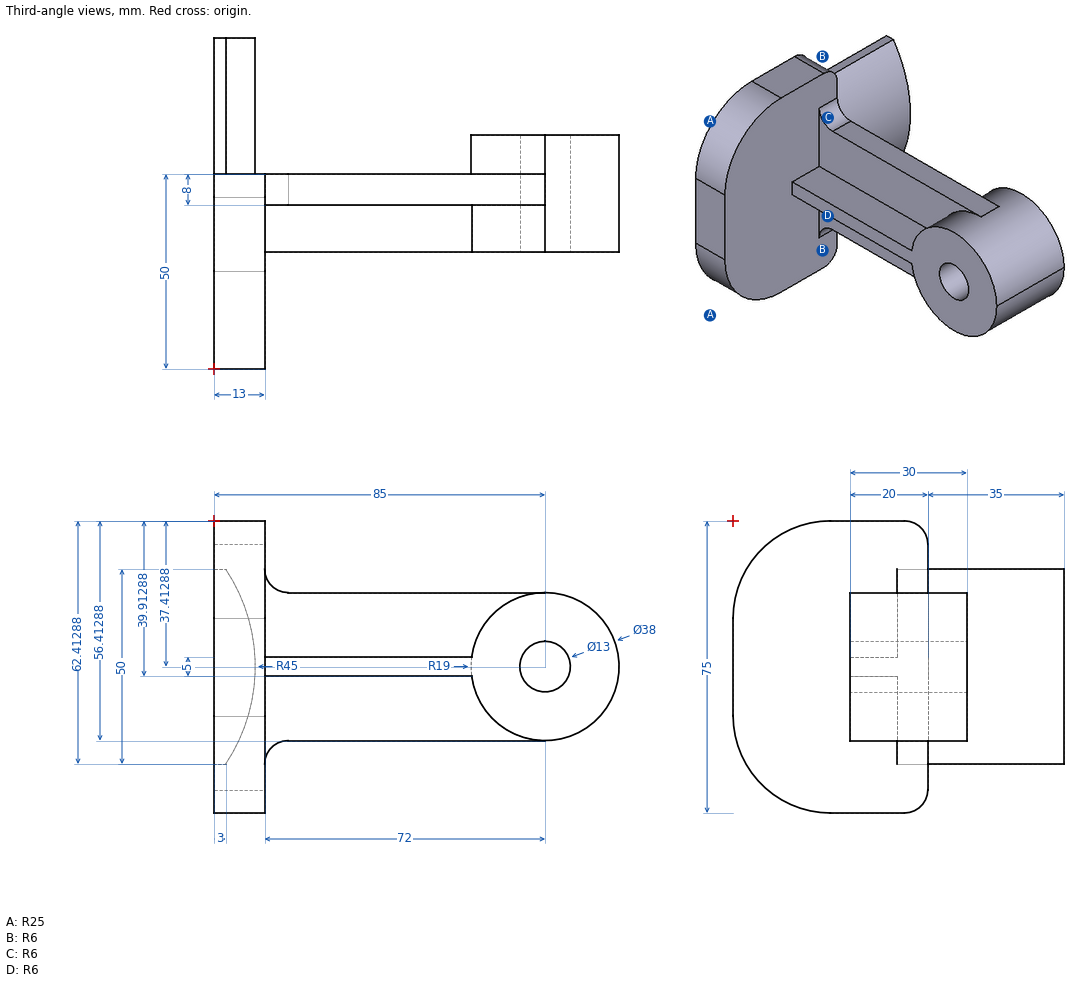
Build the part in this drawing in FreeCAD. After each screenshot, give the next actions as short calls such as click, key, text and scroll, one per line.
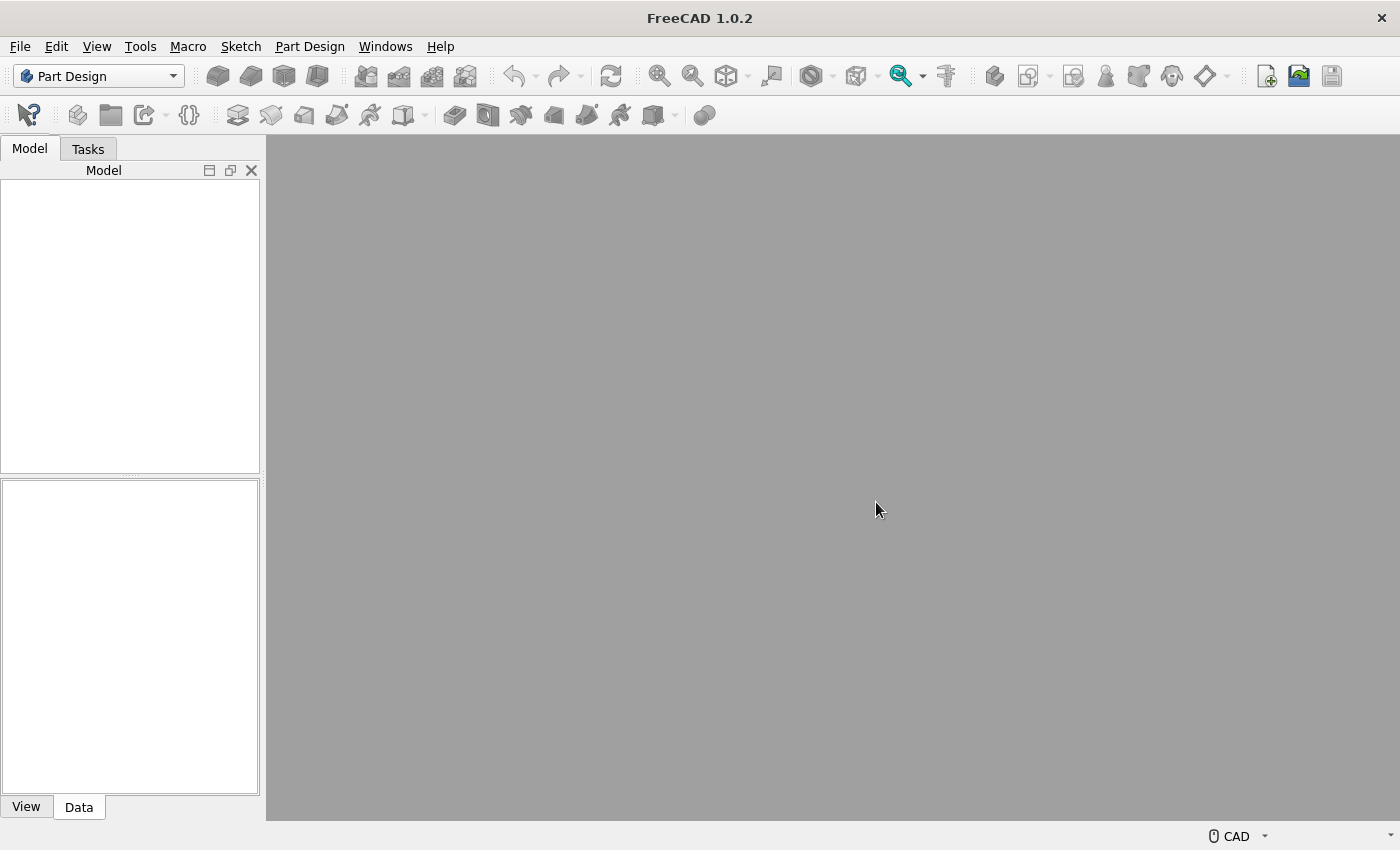
click(1266, 76)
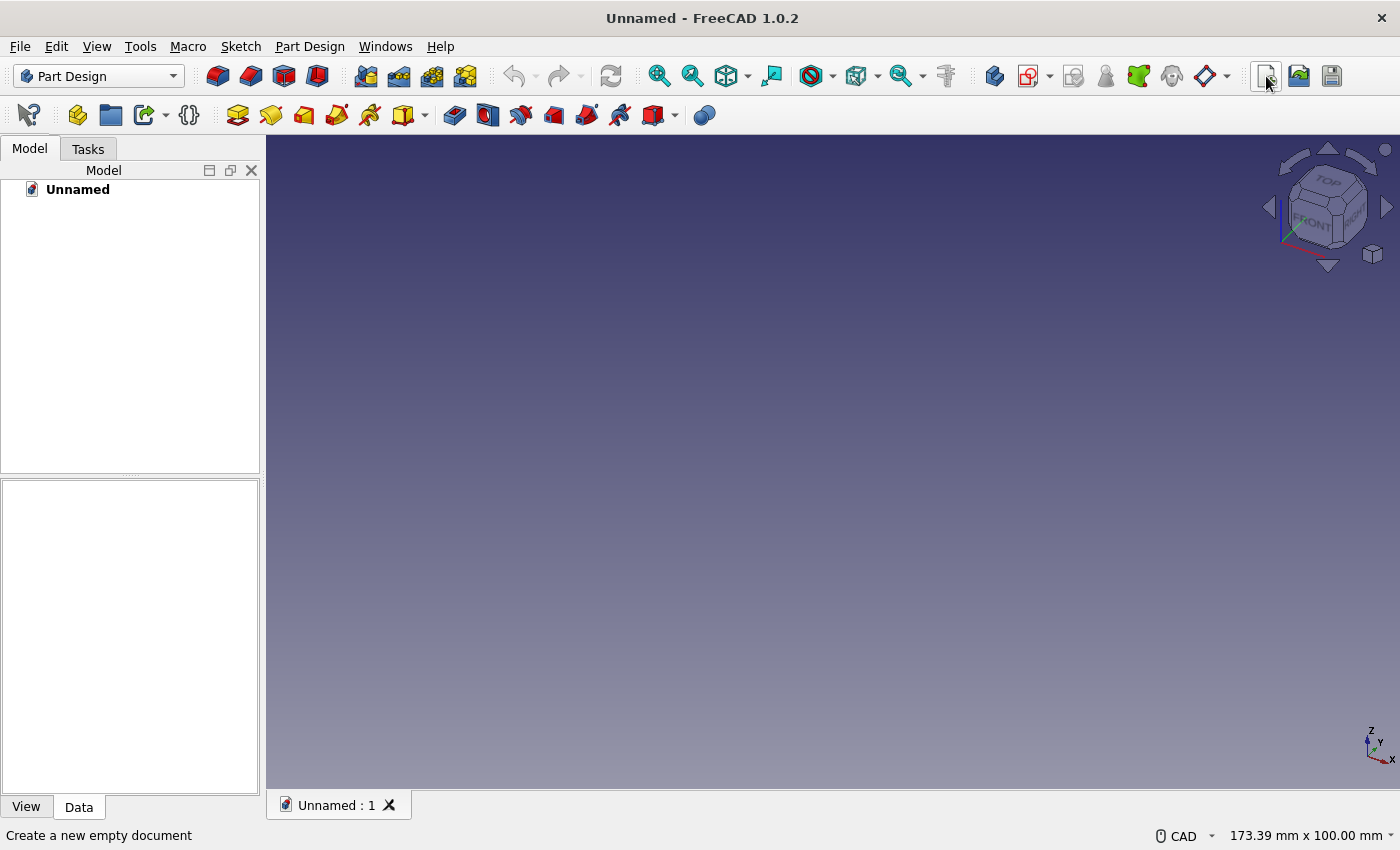
click(1028, 76)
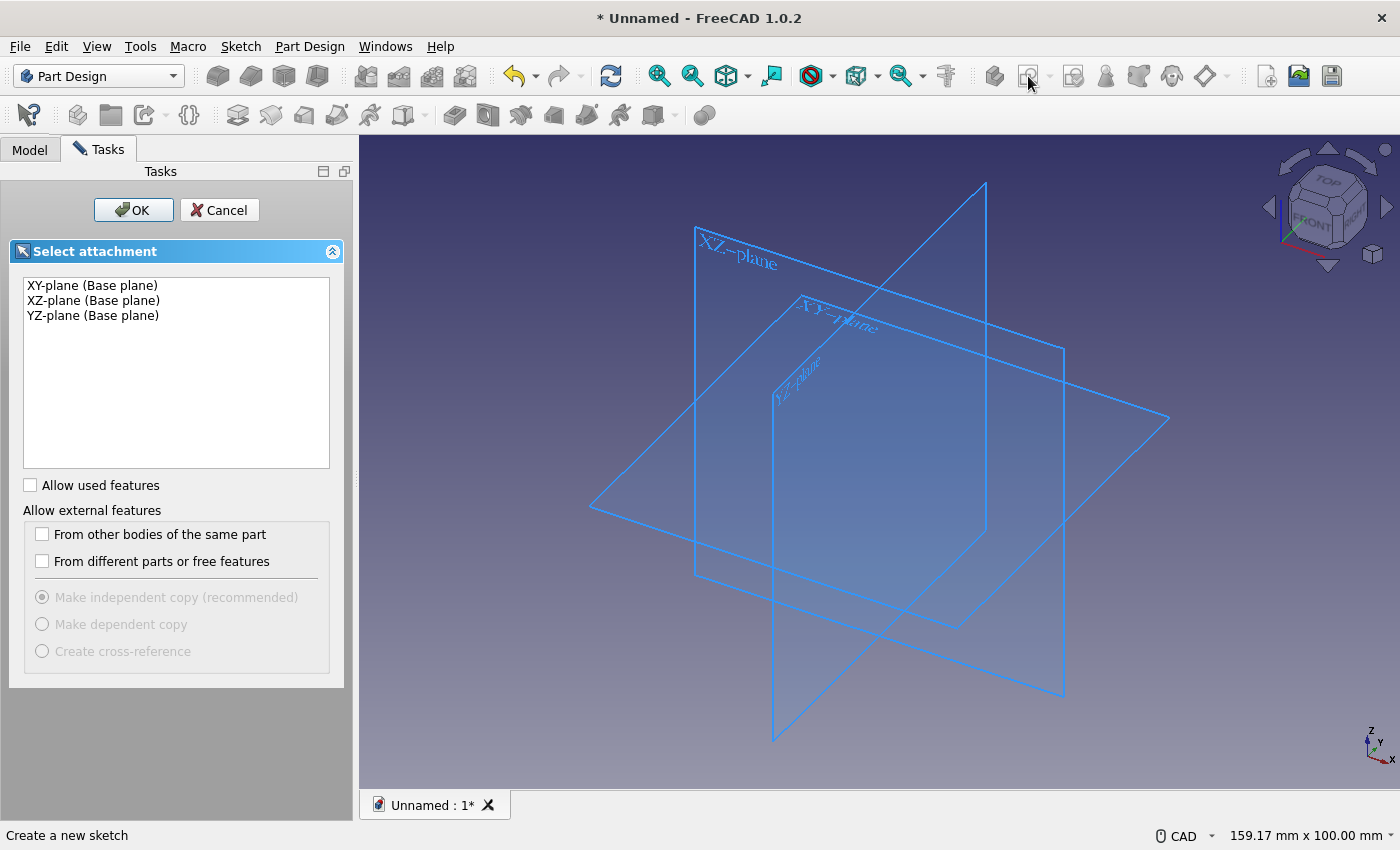
click(84, 286)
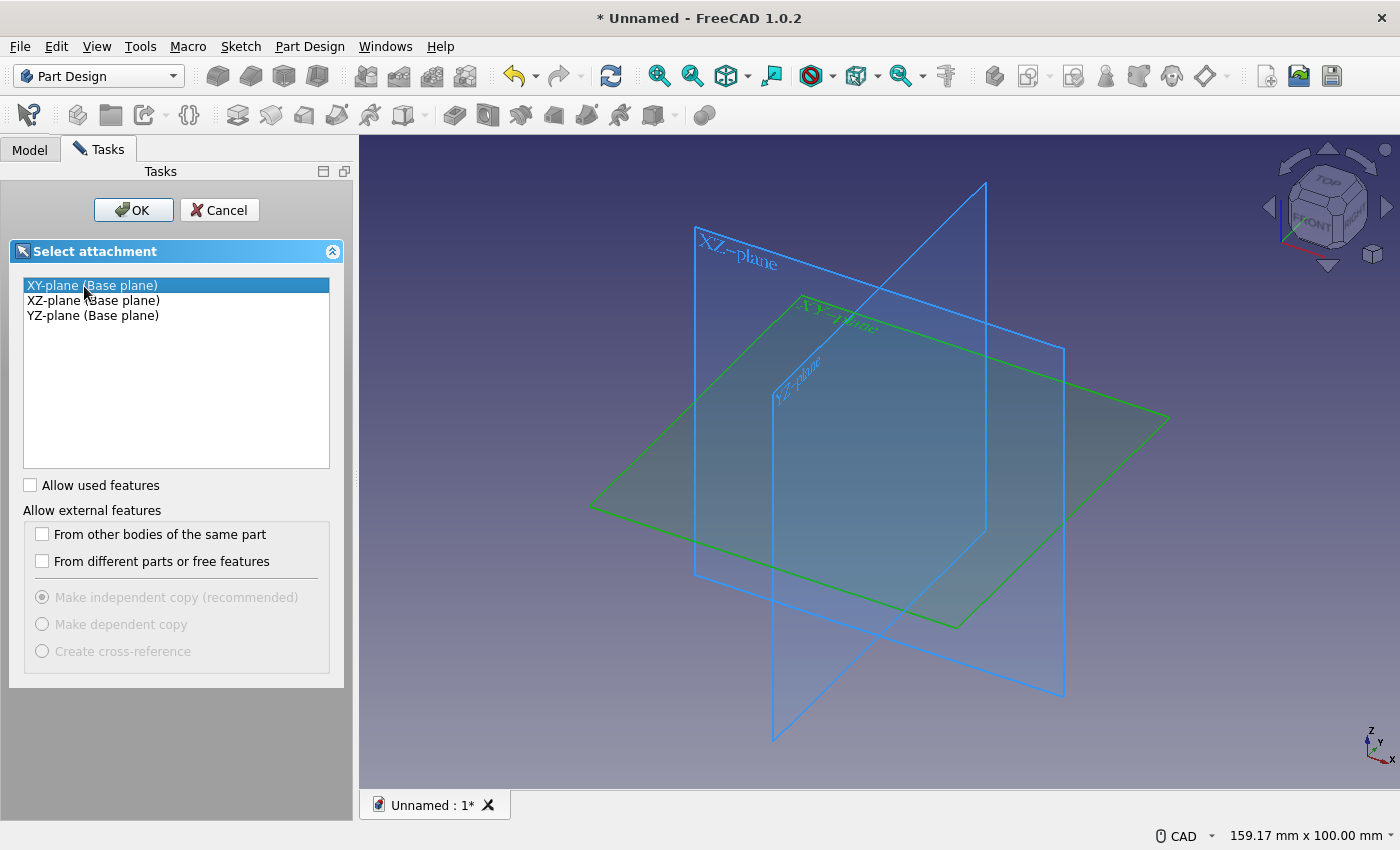
click(134, 210)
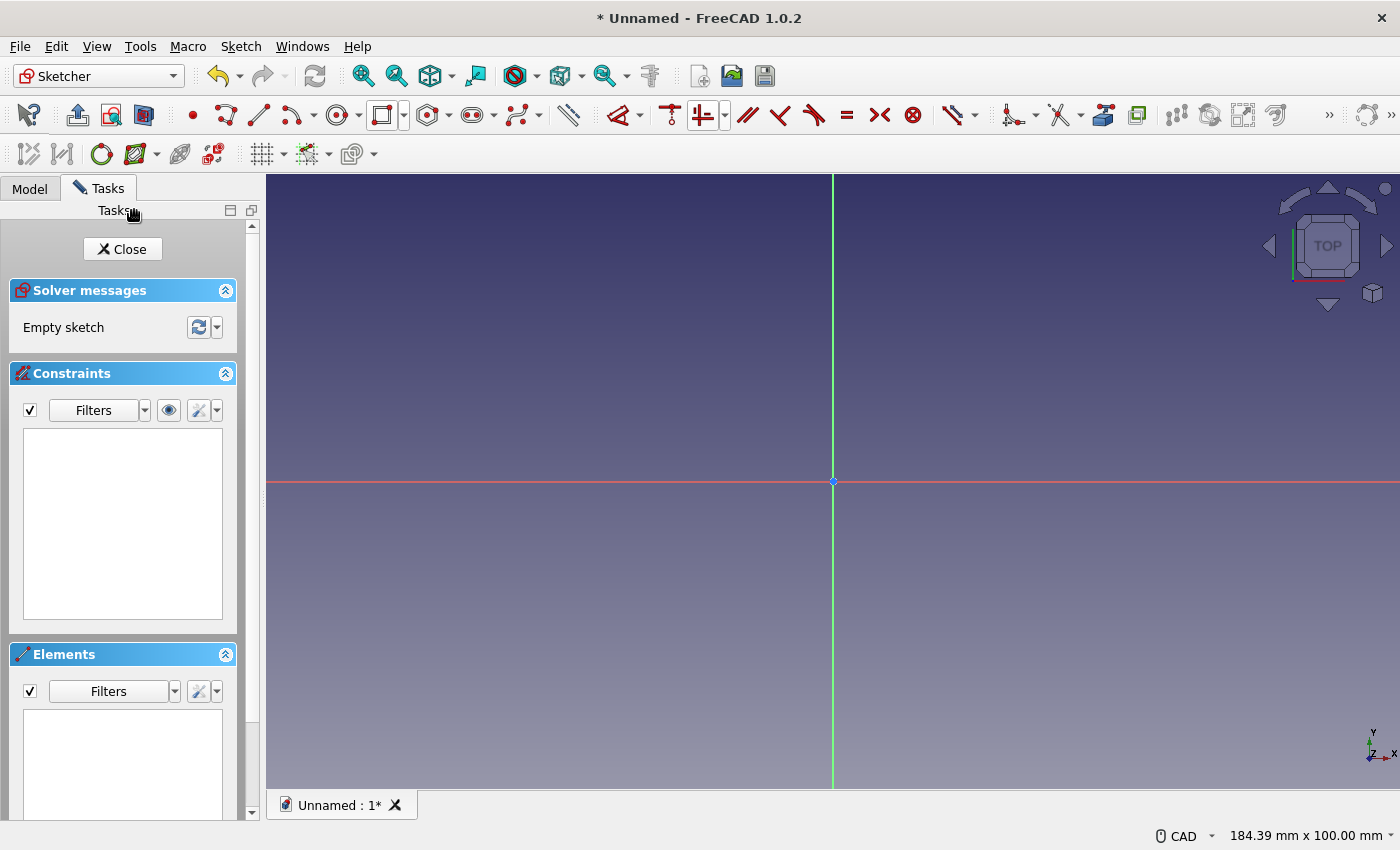
scroll(294, 761, down, 1)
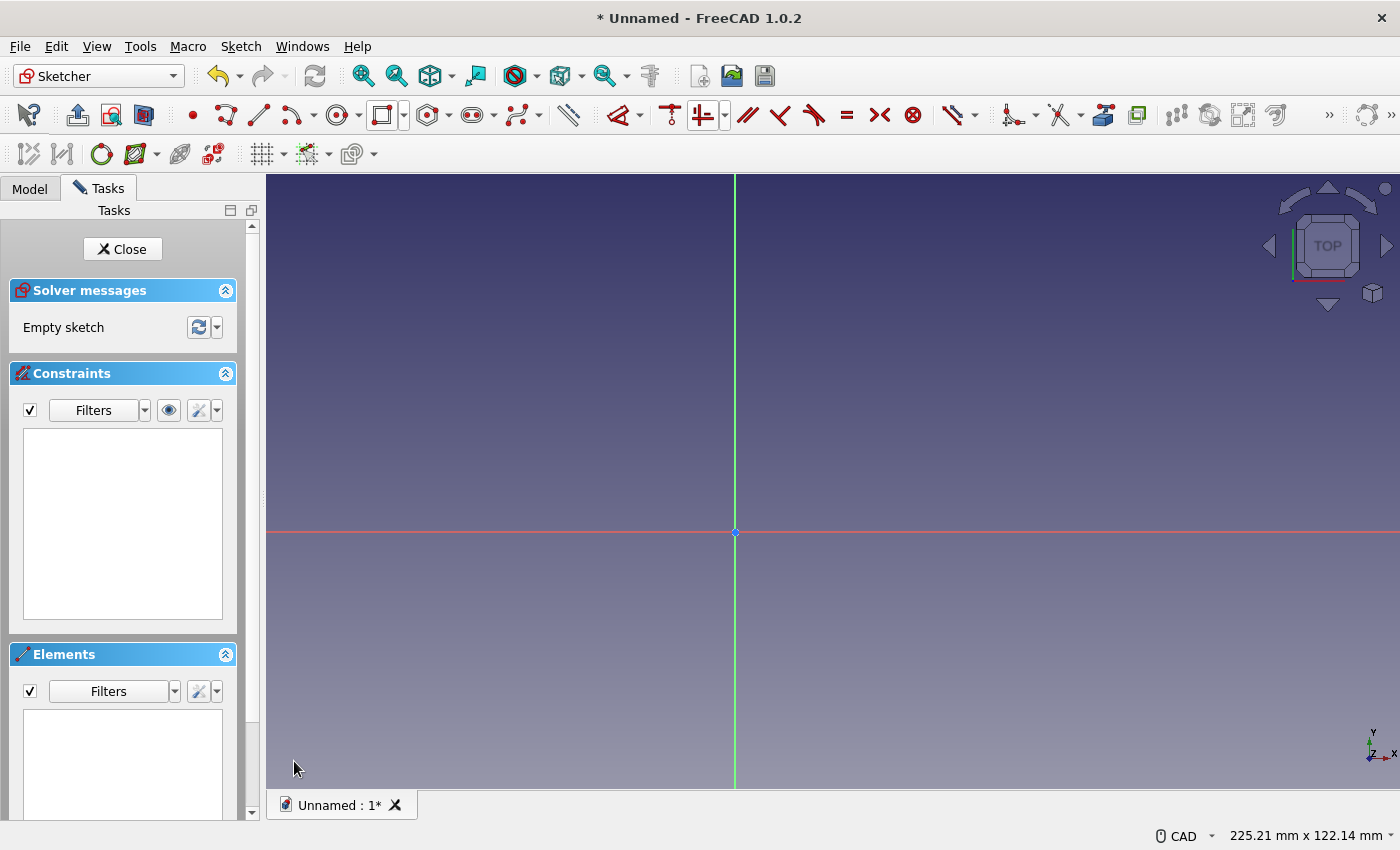
scroll(775, 254, up, 2)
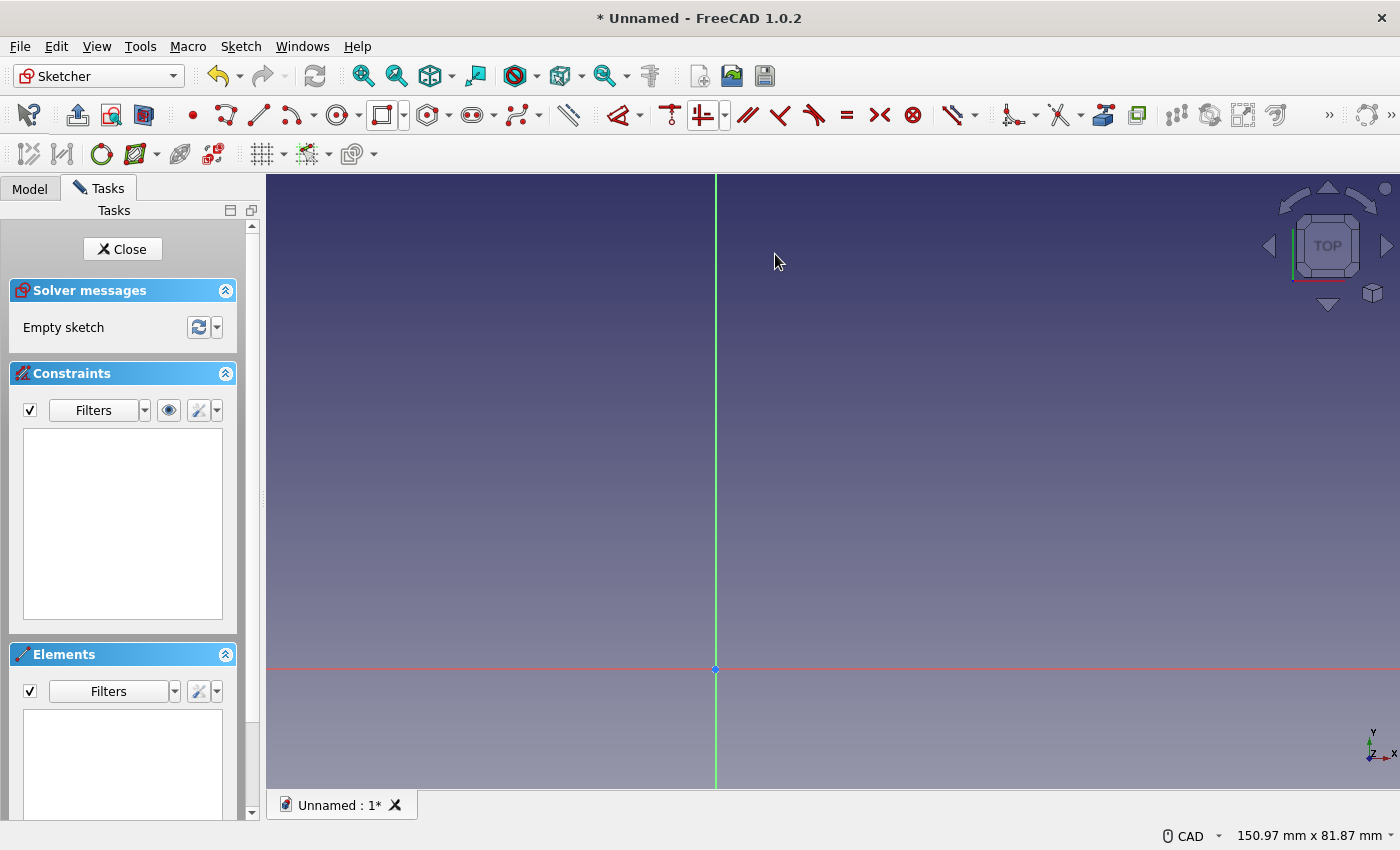
click(382, 116)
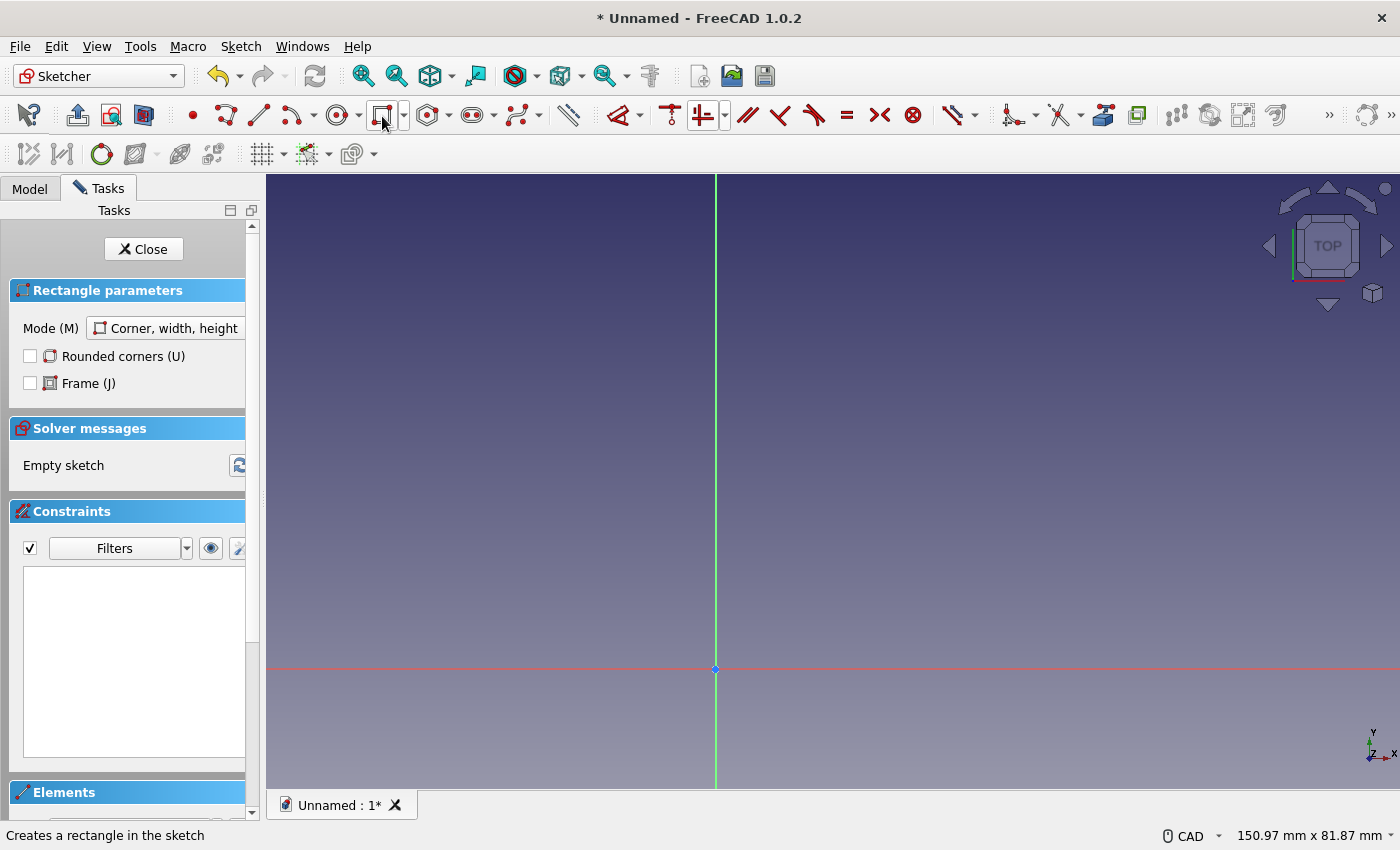
click(716, 669)
click(813, 294)
key(Escape)